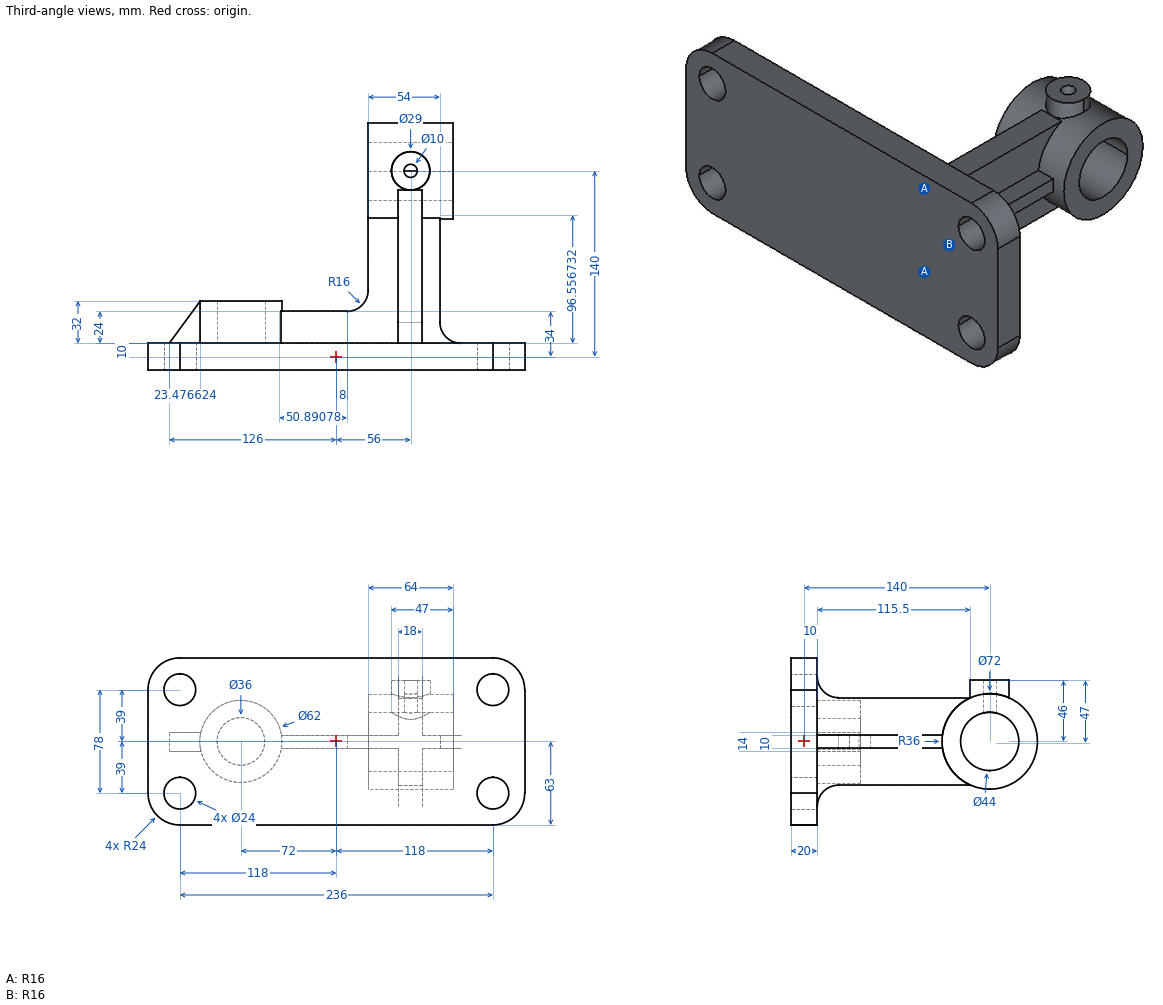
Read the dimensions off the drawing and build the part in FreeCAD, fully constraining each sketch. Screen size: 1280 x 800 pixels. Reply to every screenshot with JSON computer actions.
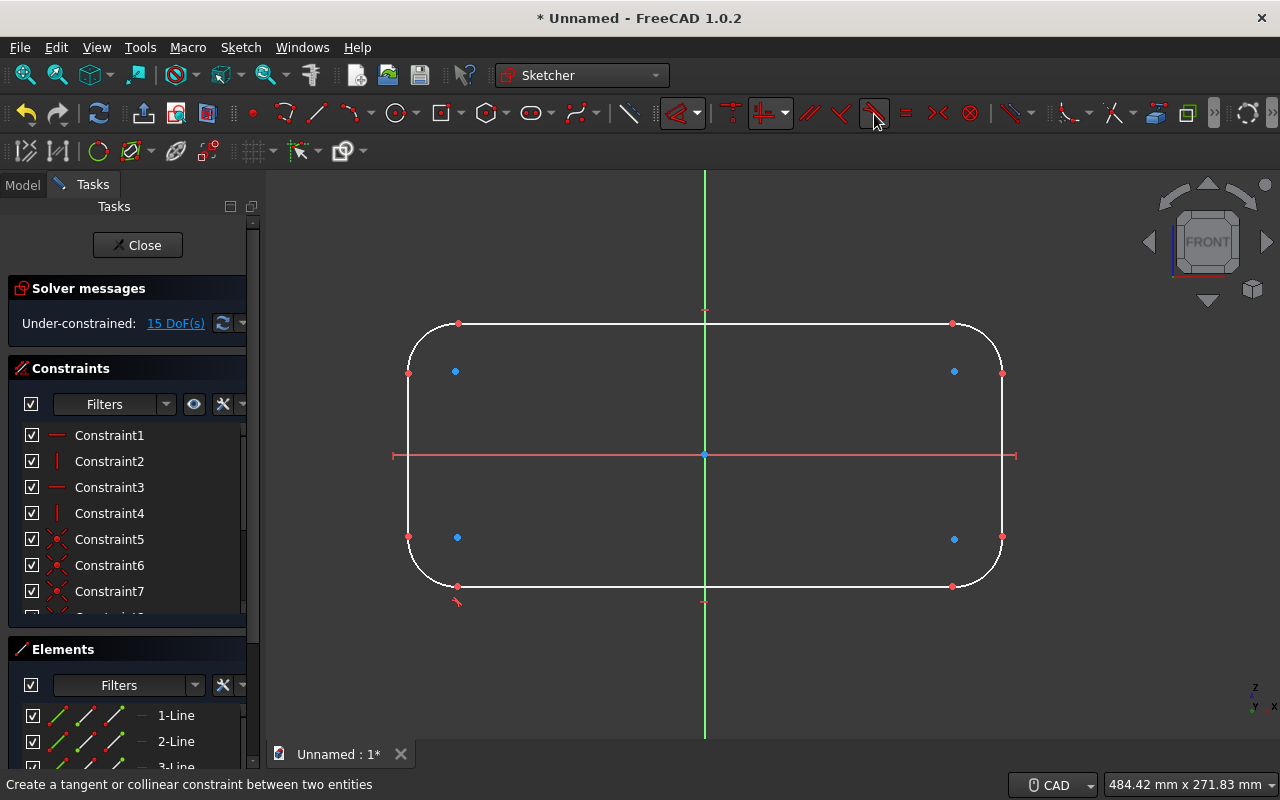
{"action": "left_click", "coordinate": [804, 587]}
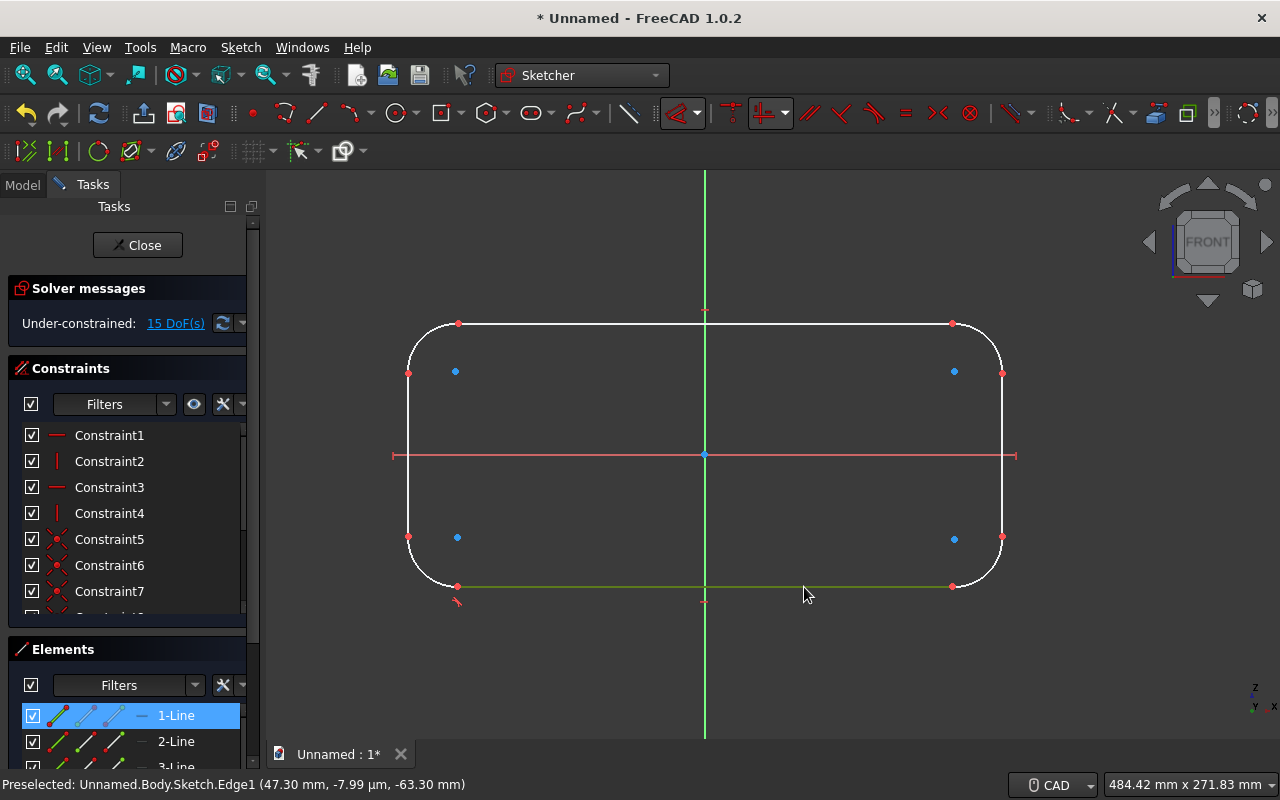
{"action": "left_click", "coordinate": [975, 582]}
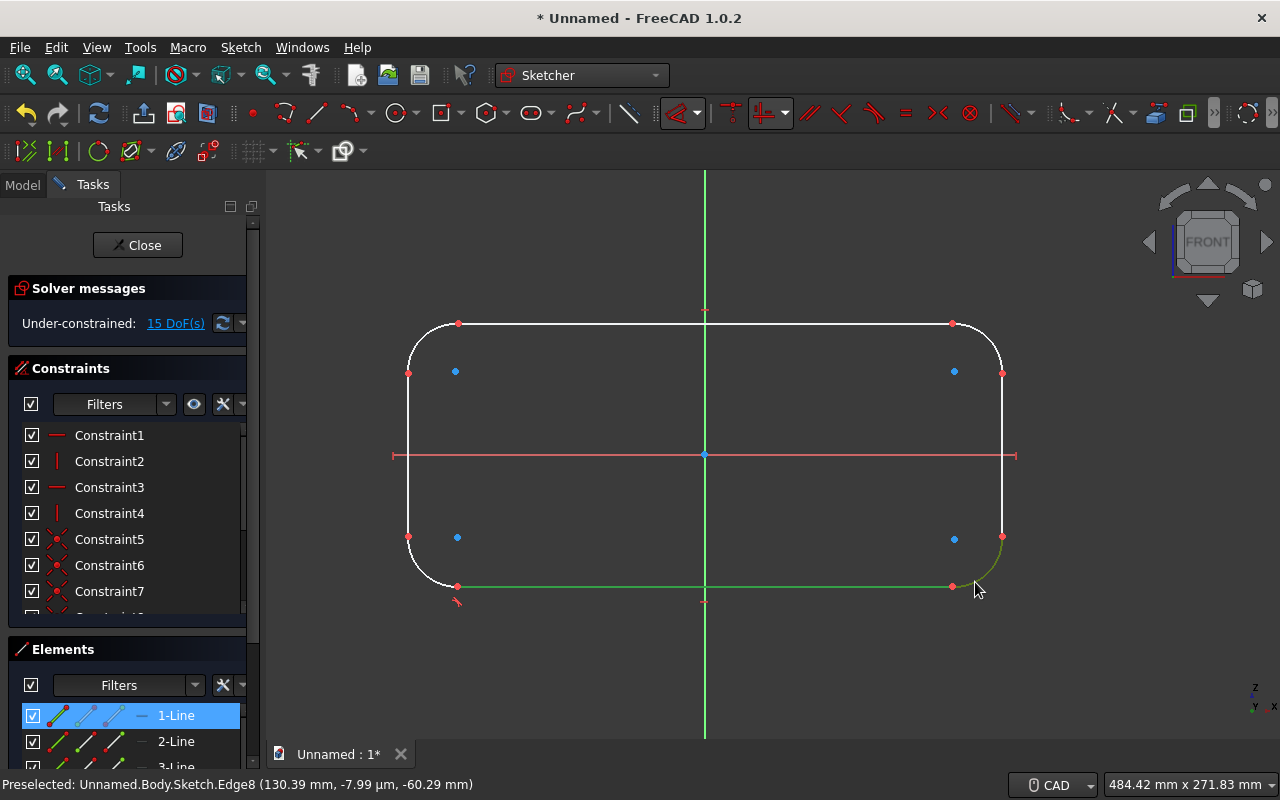
{"action": "left_click", "coordinate": [874, 114]}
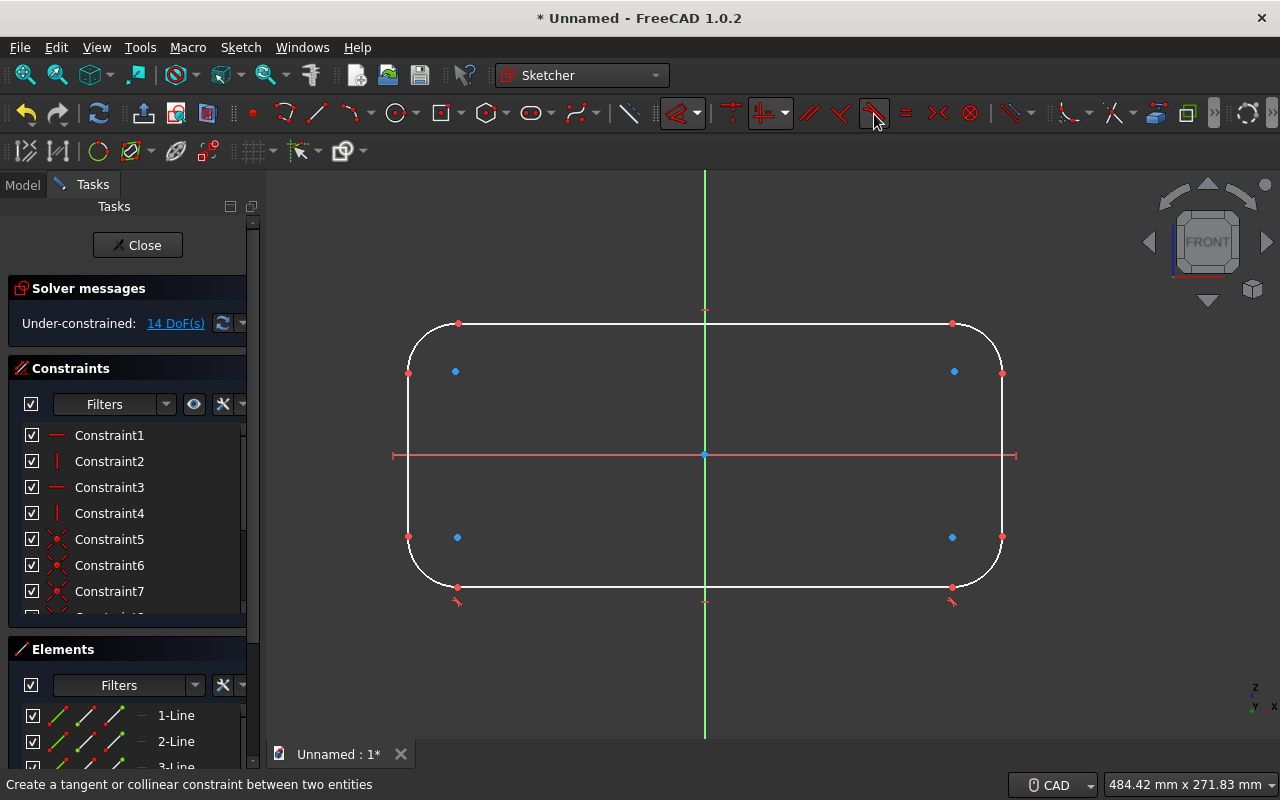
{"action": "left_click", "coordinate": [408, 488]}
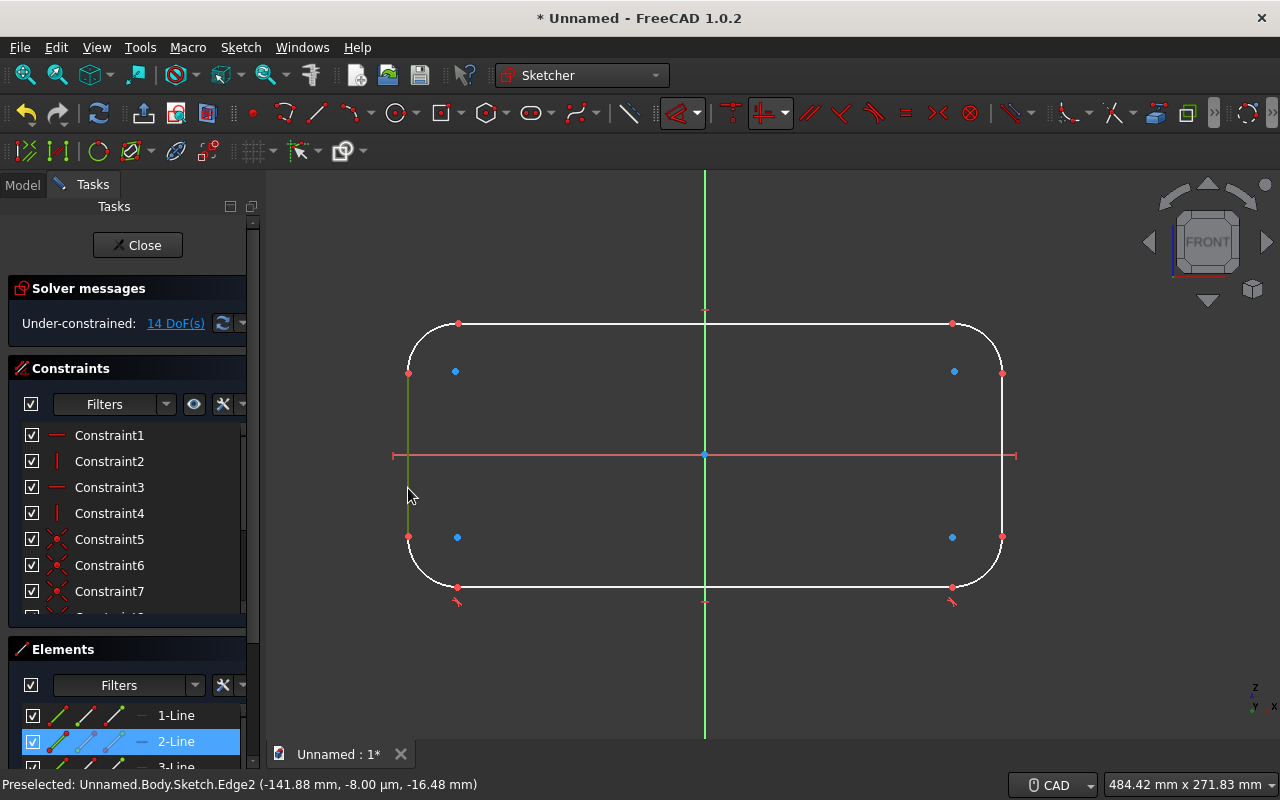
{"action": "left_click", "coordinate": [413, 560]}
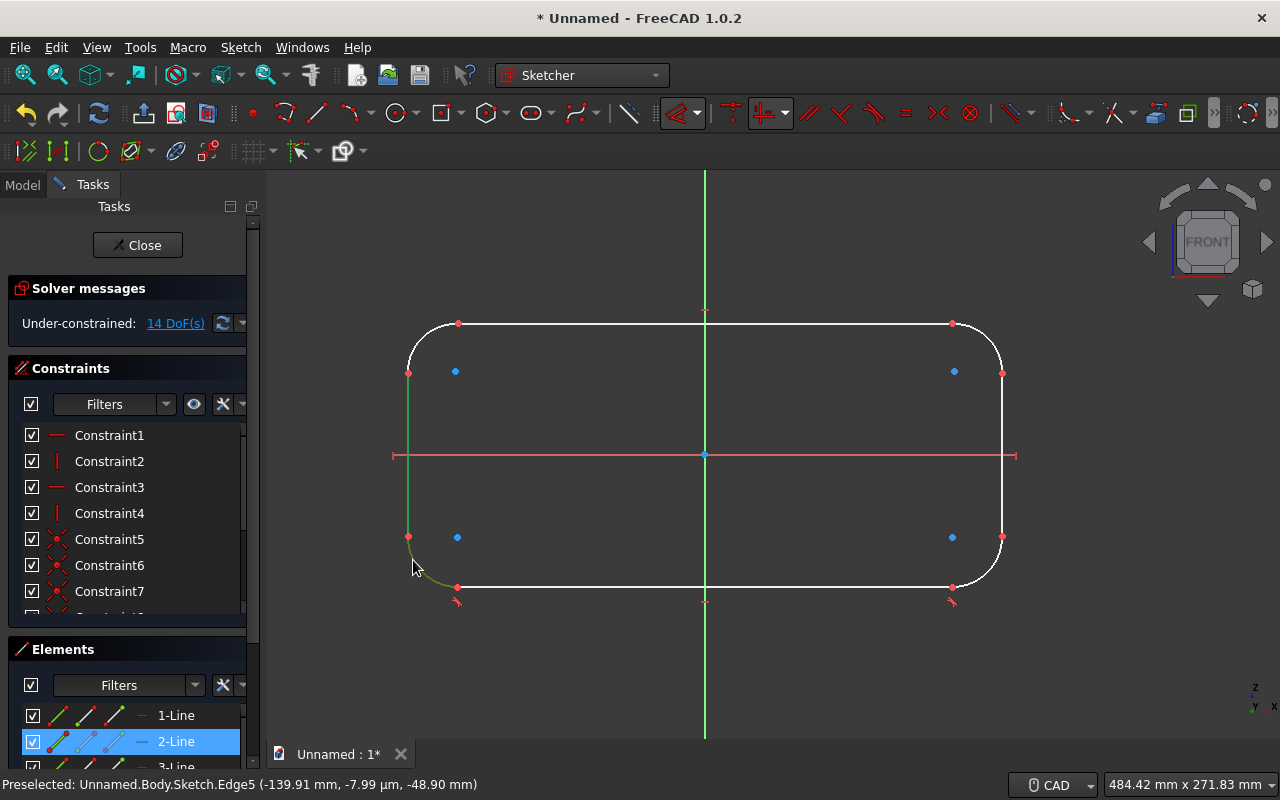
{"action": "left_click", "coordinate": [874, 114]}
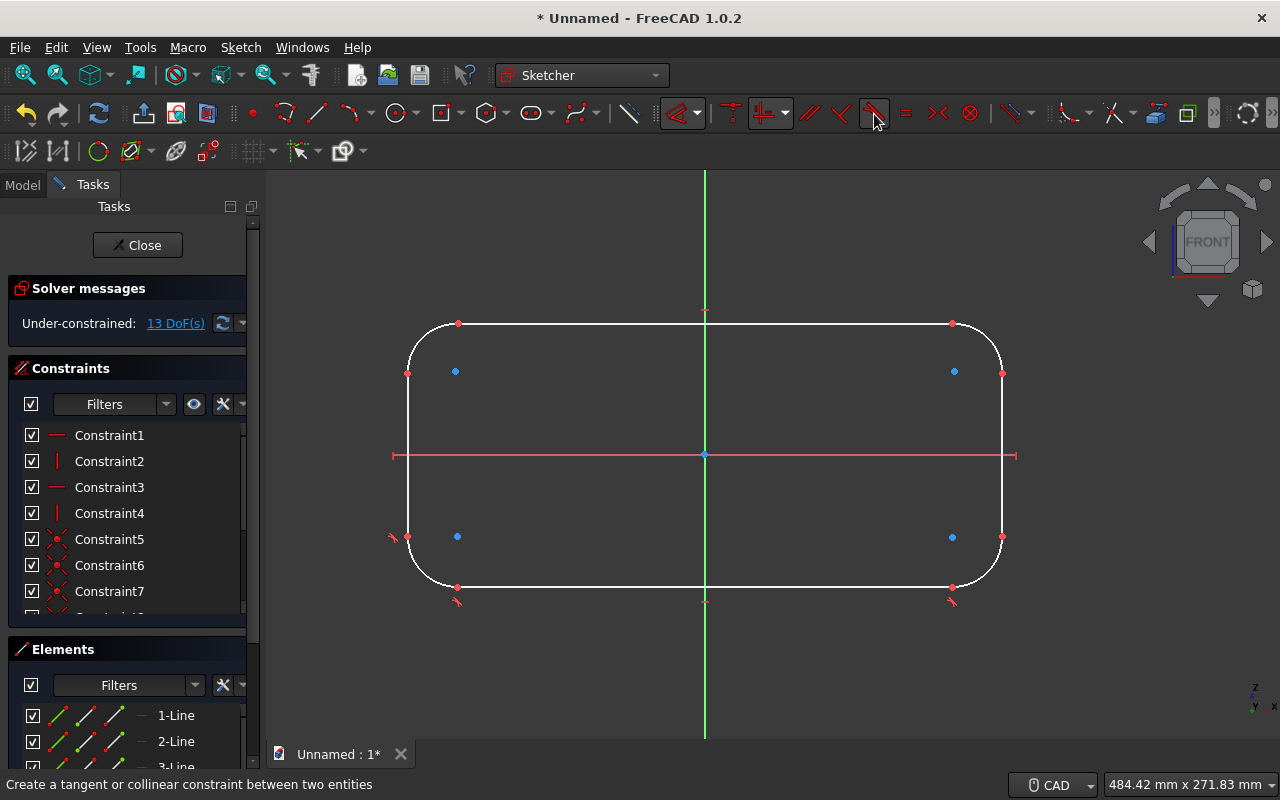
{"action": "left_click", "coordinate": [408, 488]}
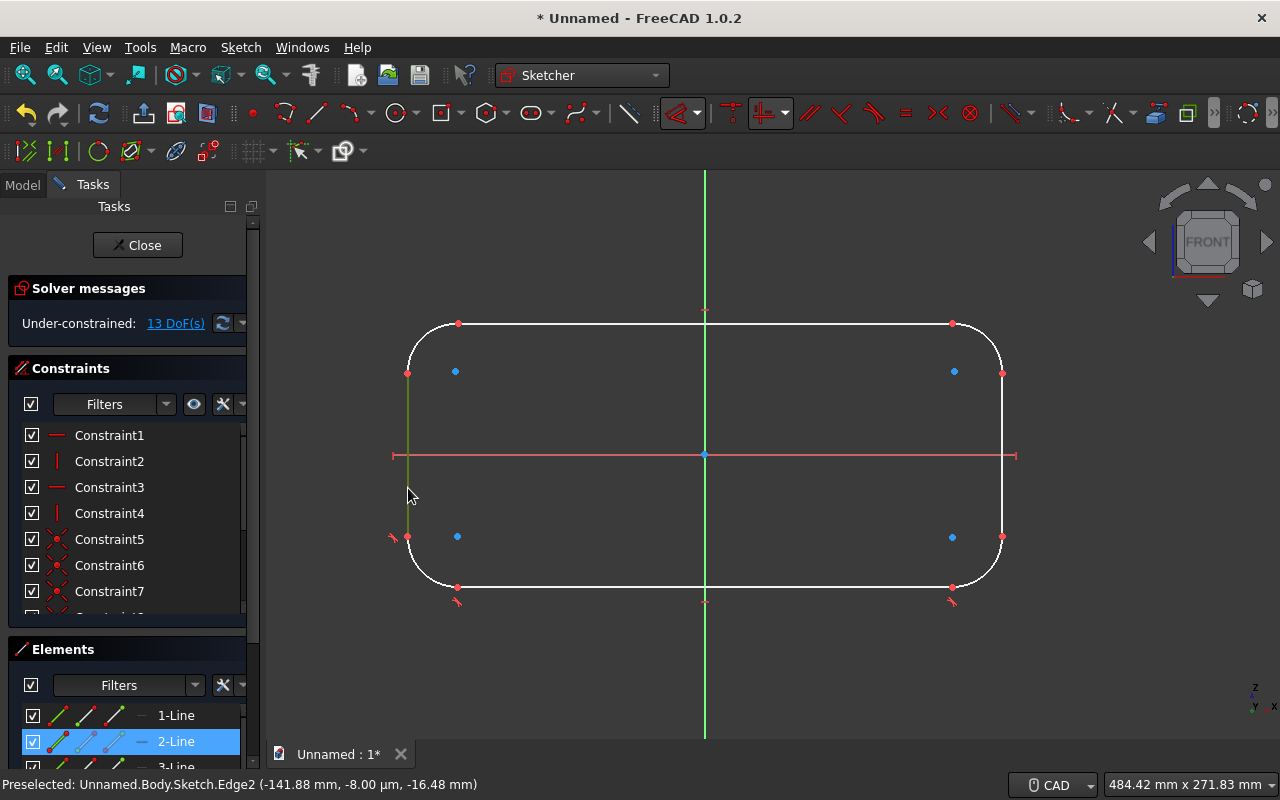
{"action": "left_click", "coordinate": [435, 329]}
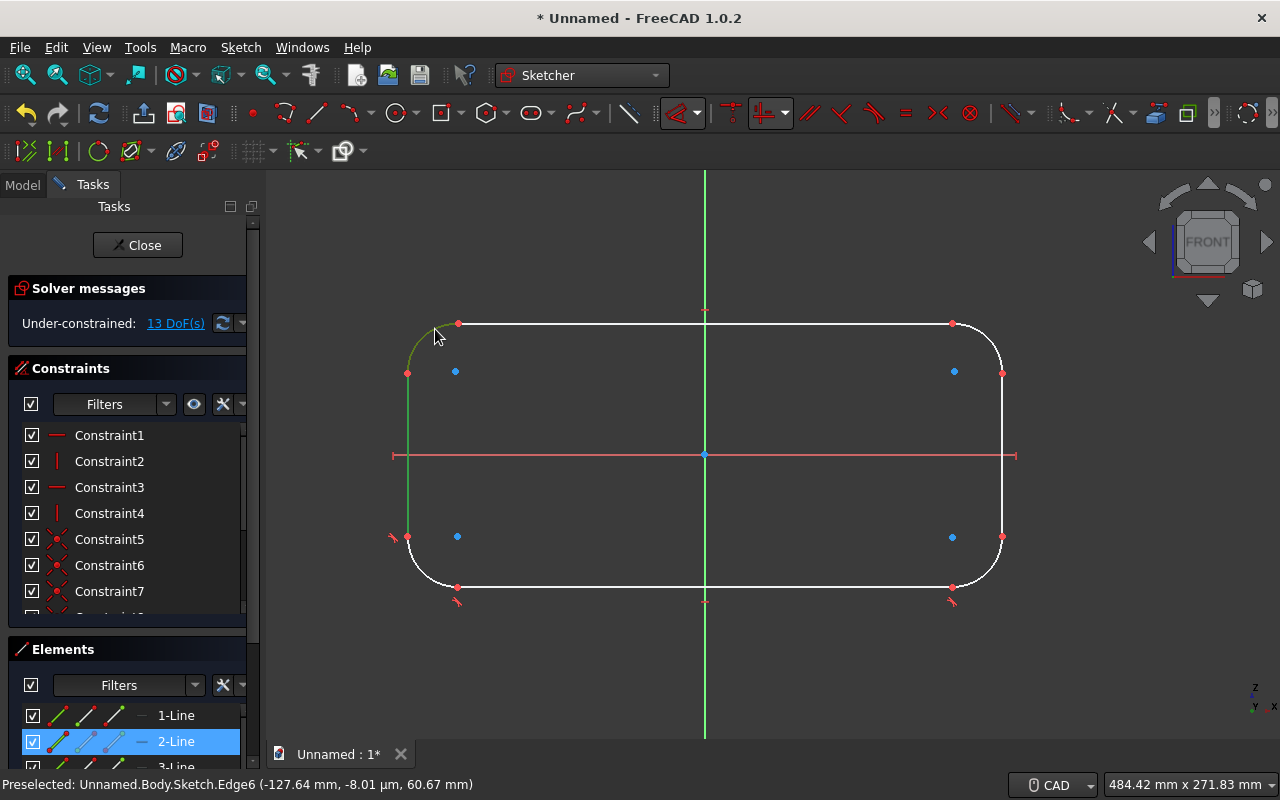
{"action": "left_click", "coordinate": [874, 114]}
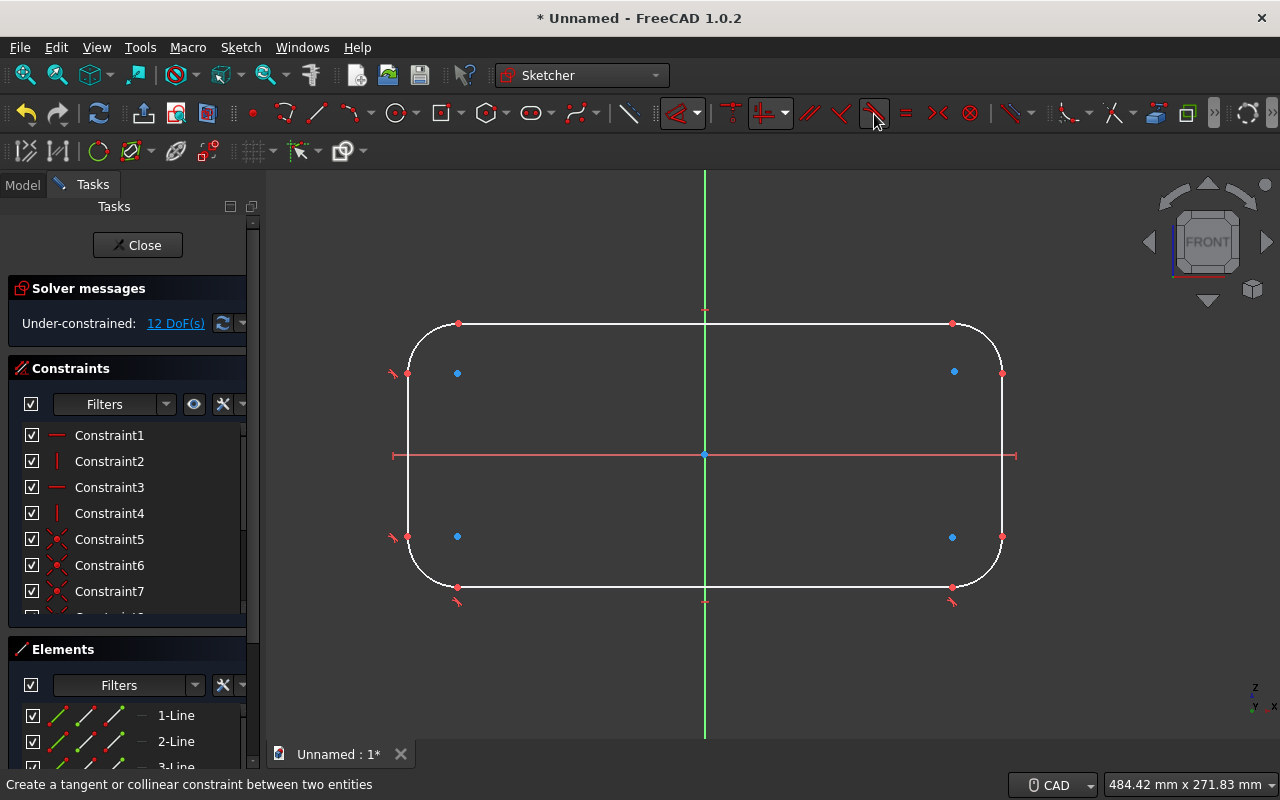
{"action": "left_click", "coordinate": [606, 324]}